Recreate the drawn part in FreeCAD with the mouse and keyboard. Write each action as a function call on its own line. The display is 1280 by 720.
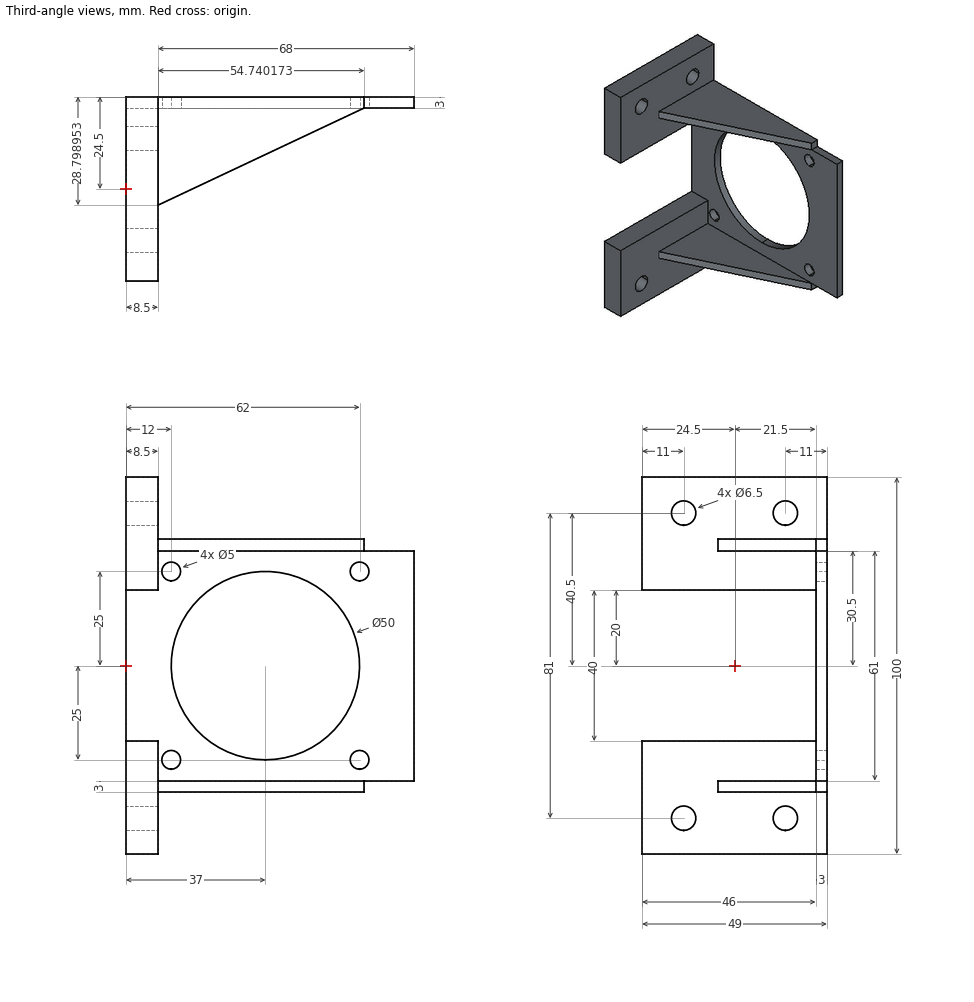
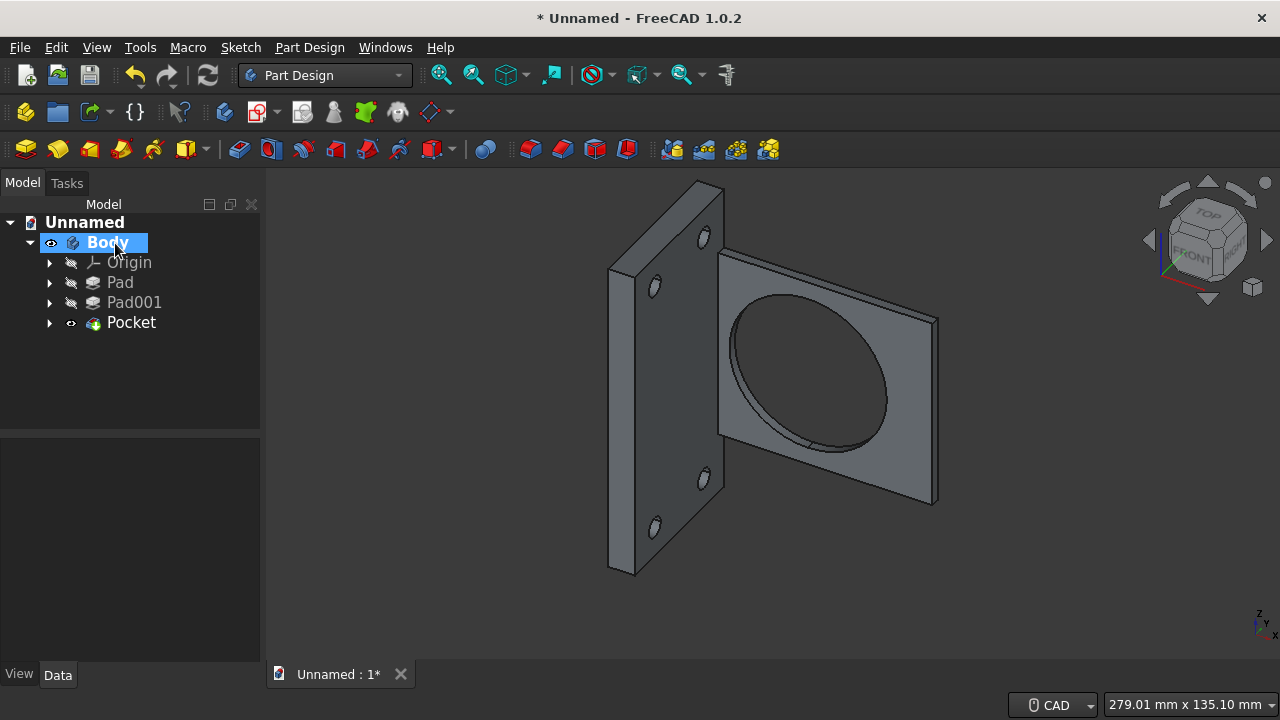
click(887, 450)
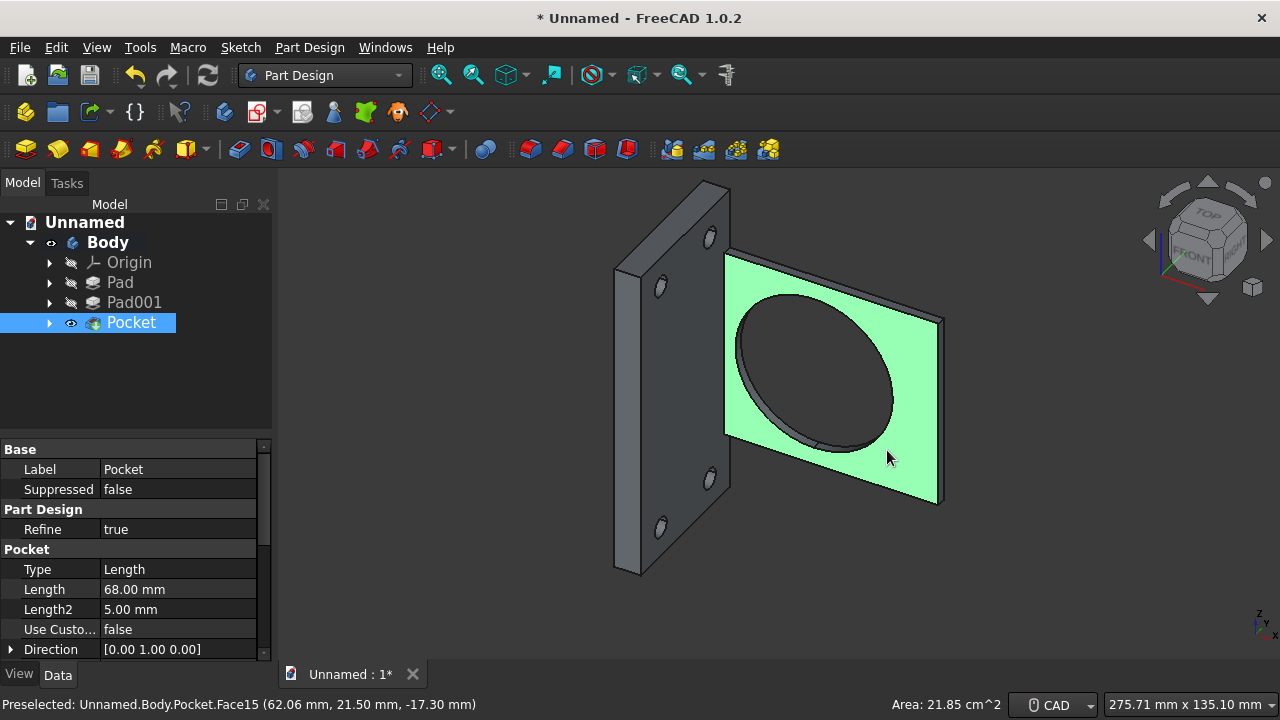
click(258, 112)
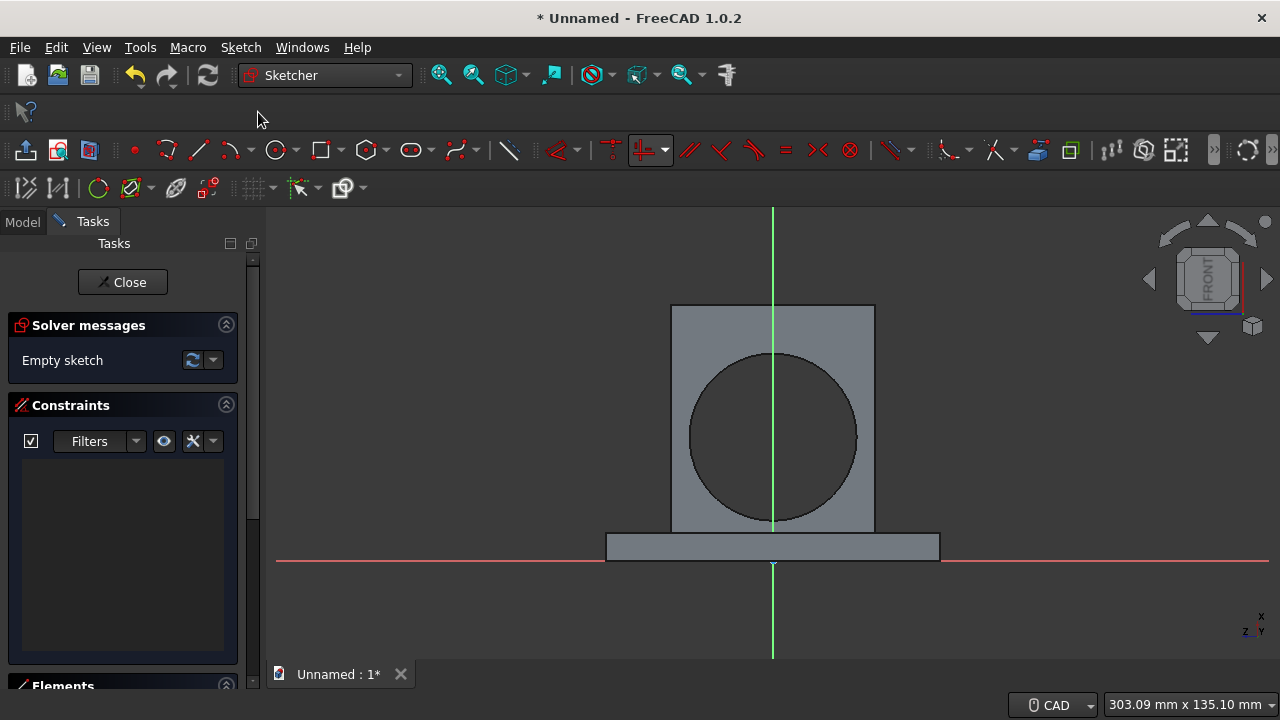
click(276, 150)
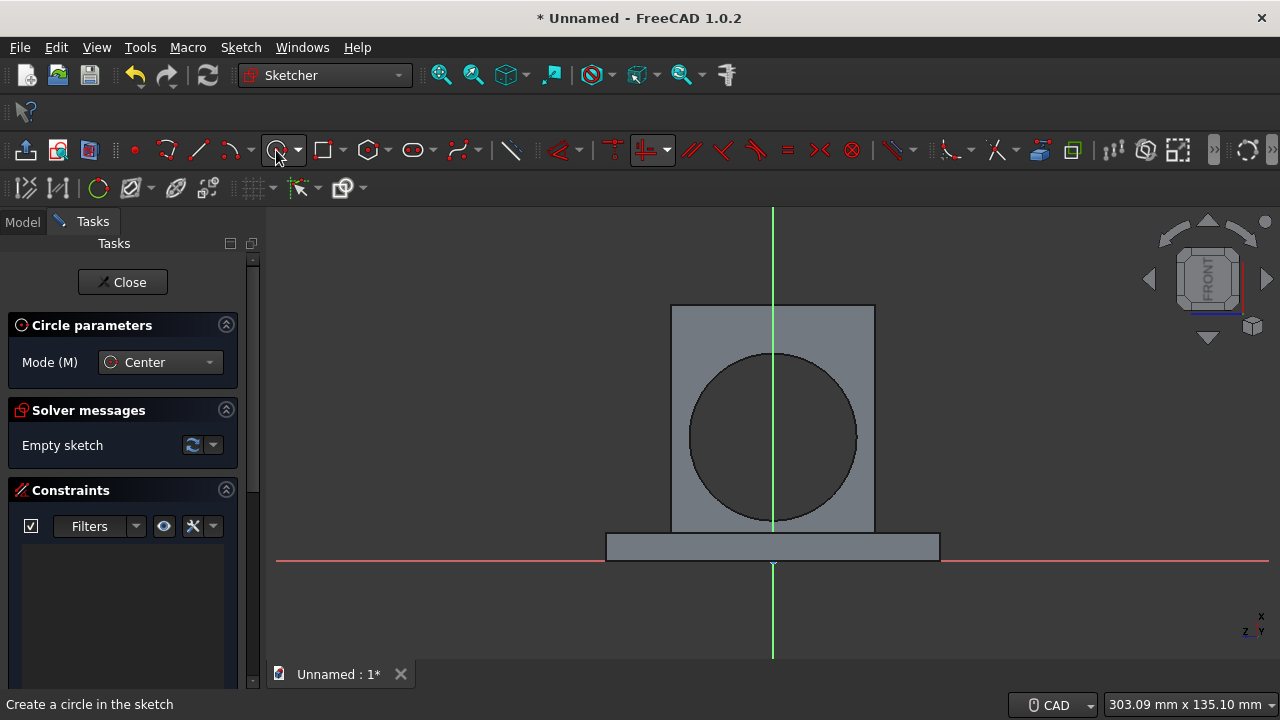
scroll(689, 521, up, 5)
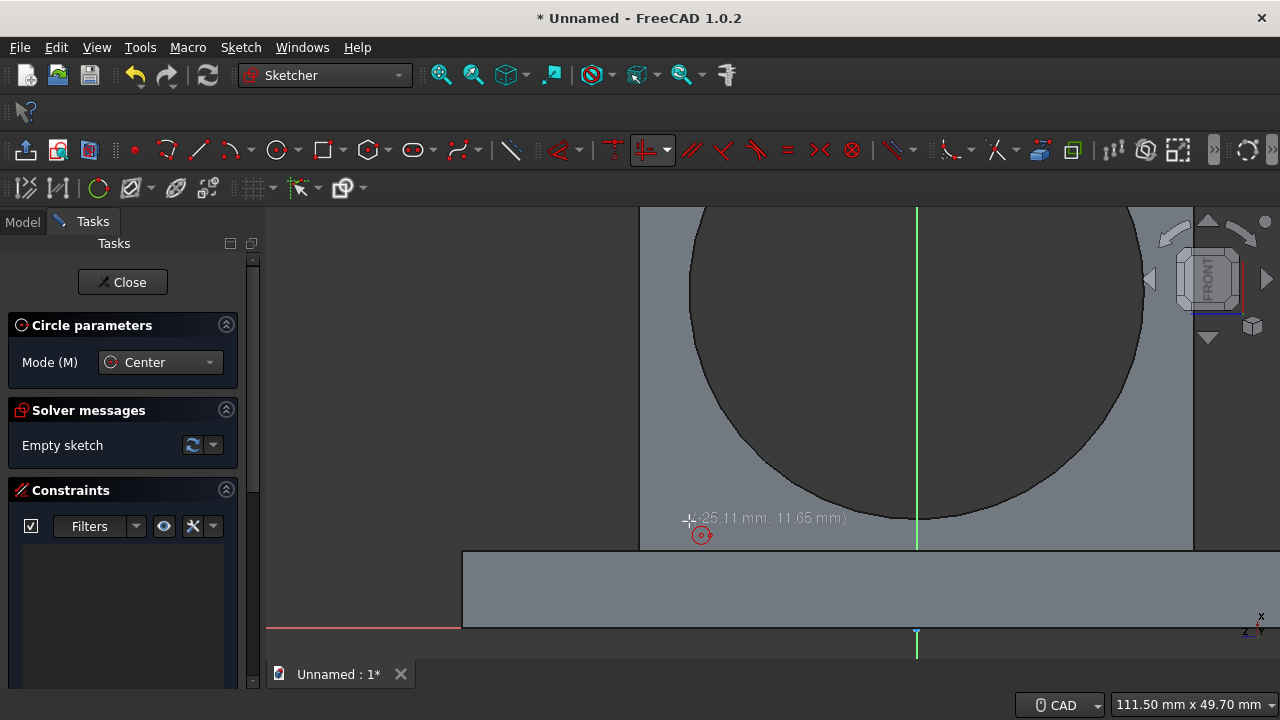
click(689, 519)
click(705, 503)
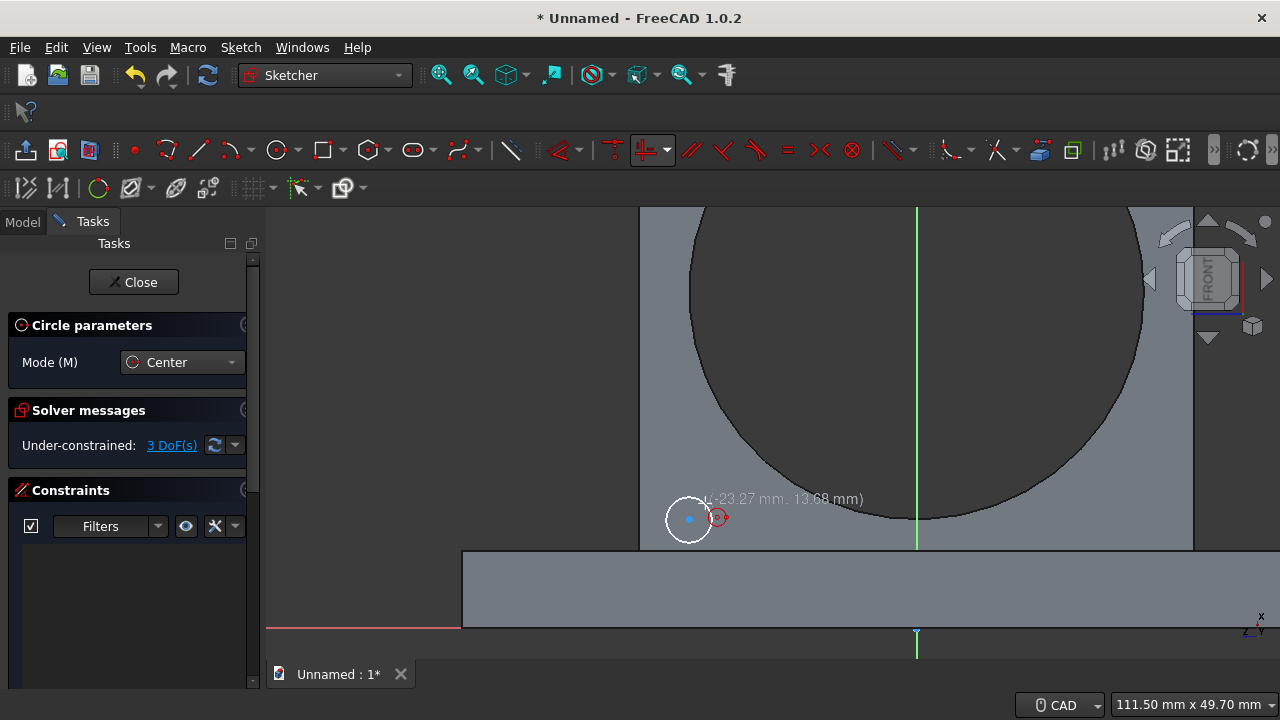
scroll(531, 513, down, 4)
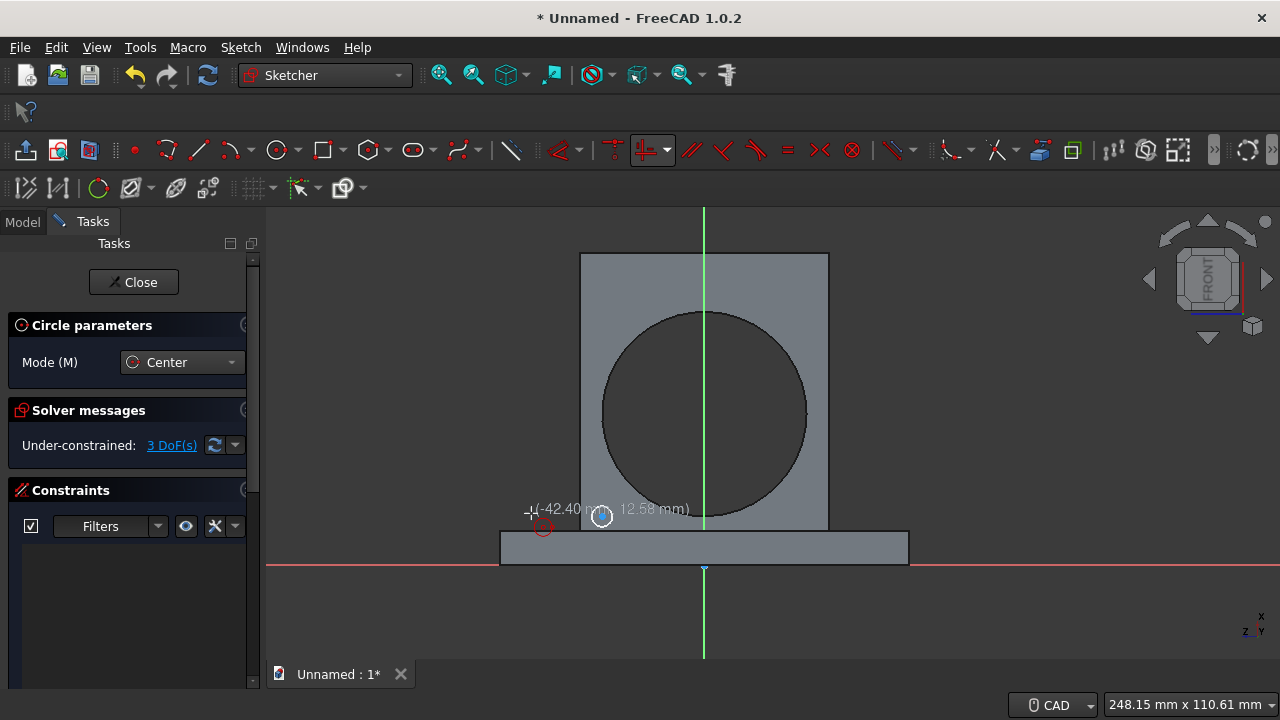
scroll(602, 312, up, 4)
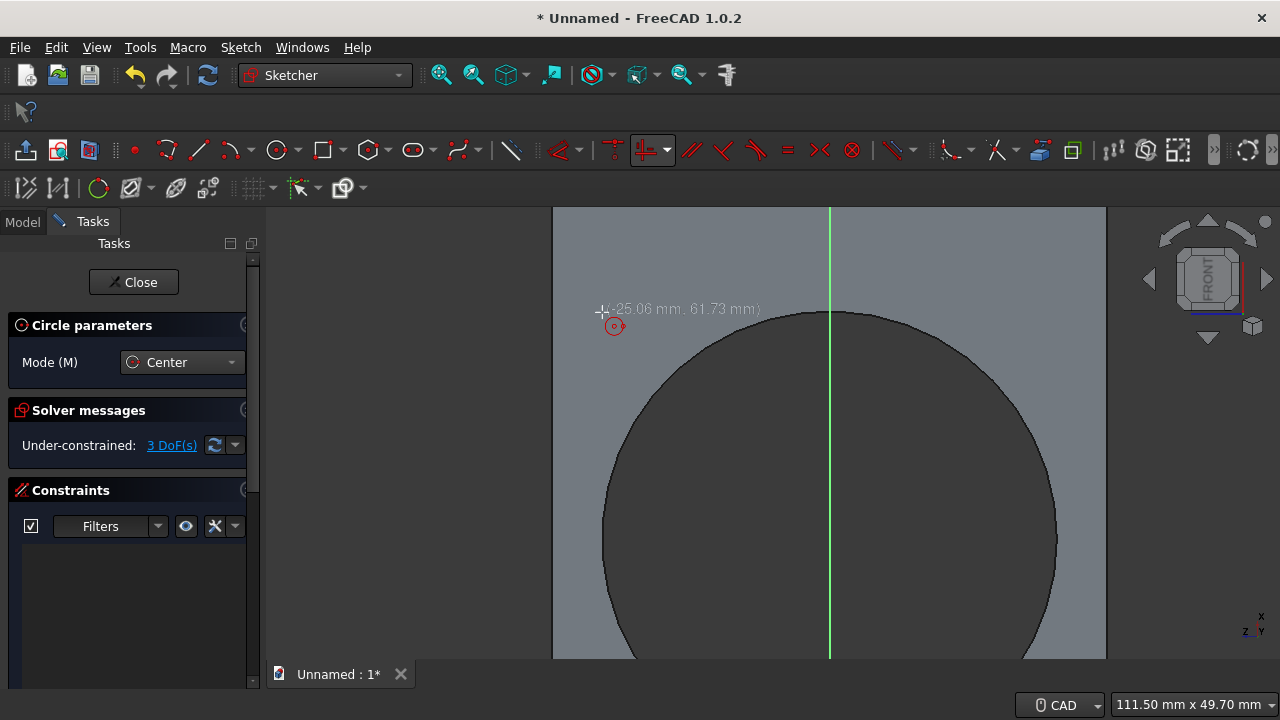
click(602, 311)
click(618, 295)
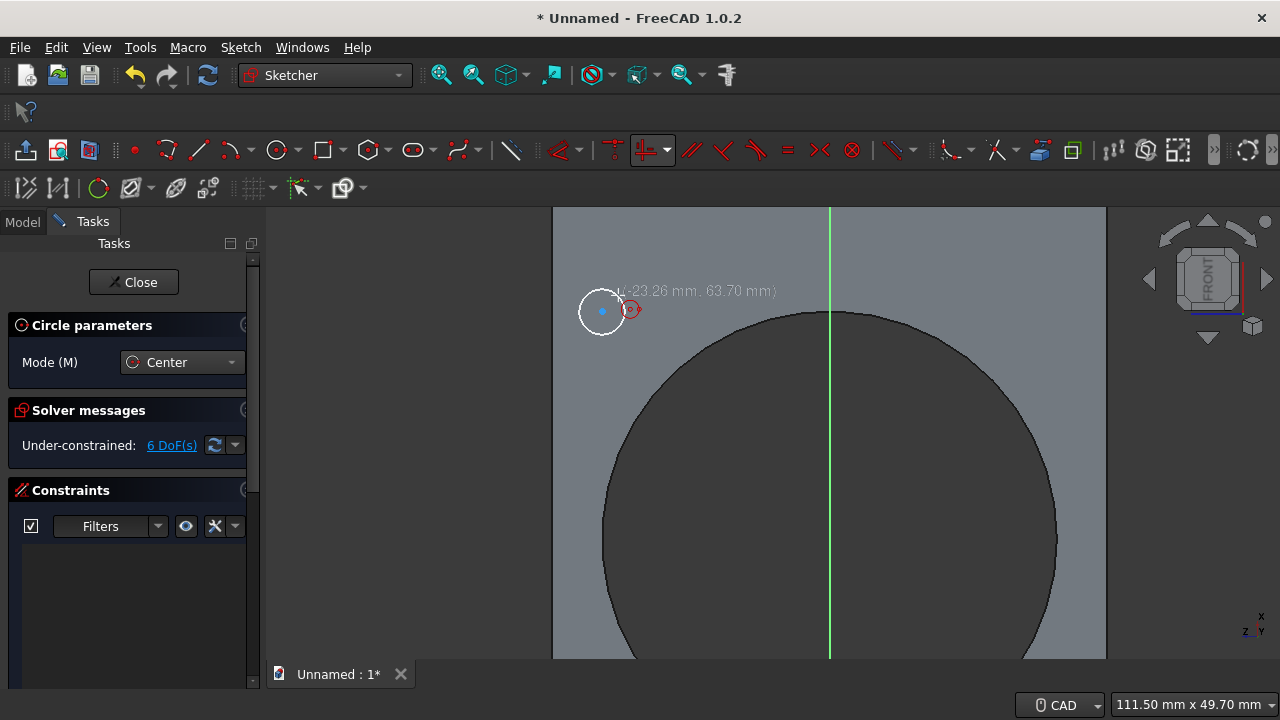
click(1057, 311)
click(1073, 295)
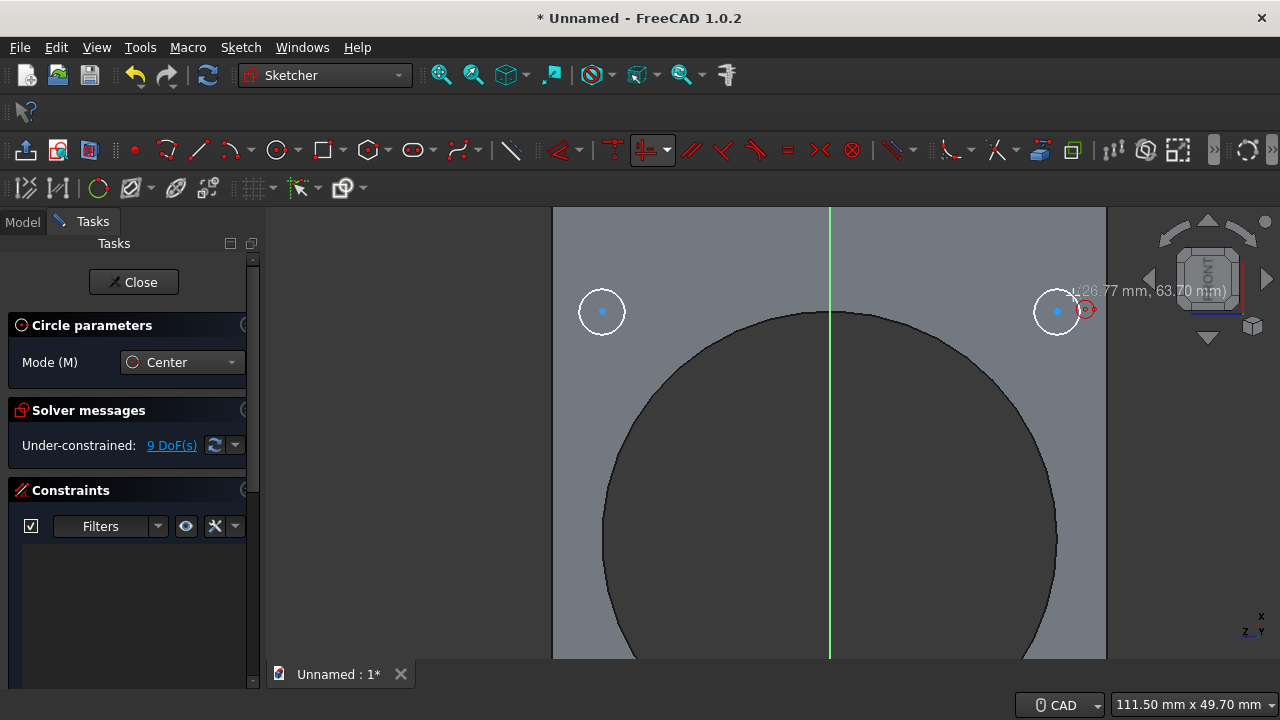
scroll(602, 311, down, 4)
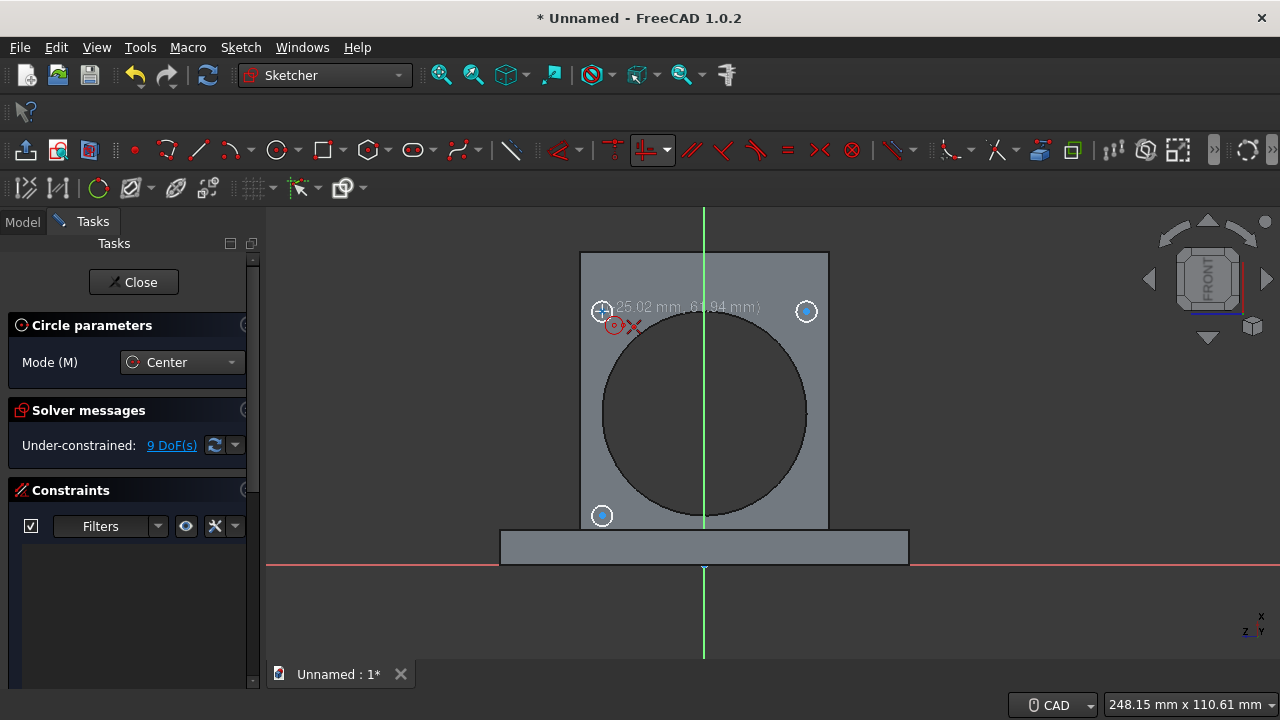
scroll(807, 516, up, 4)